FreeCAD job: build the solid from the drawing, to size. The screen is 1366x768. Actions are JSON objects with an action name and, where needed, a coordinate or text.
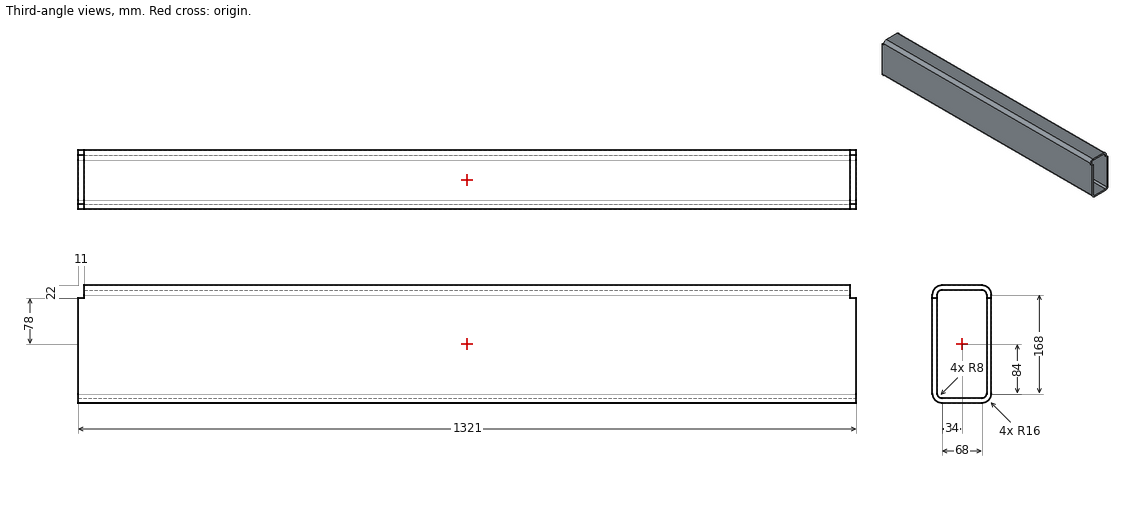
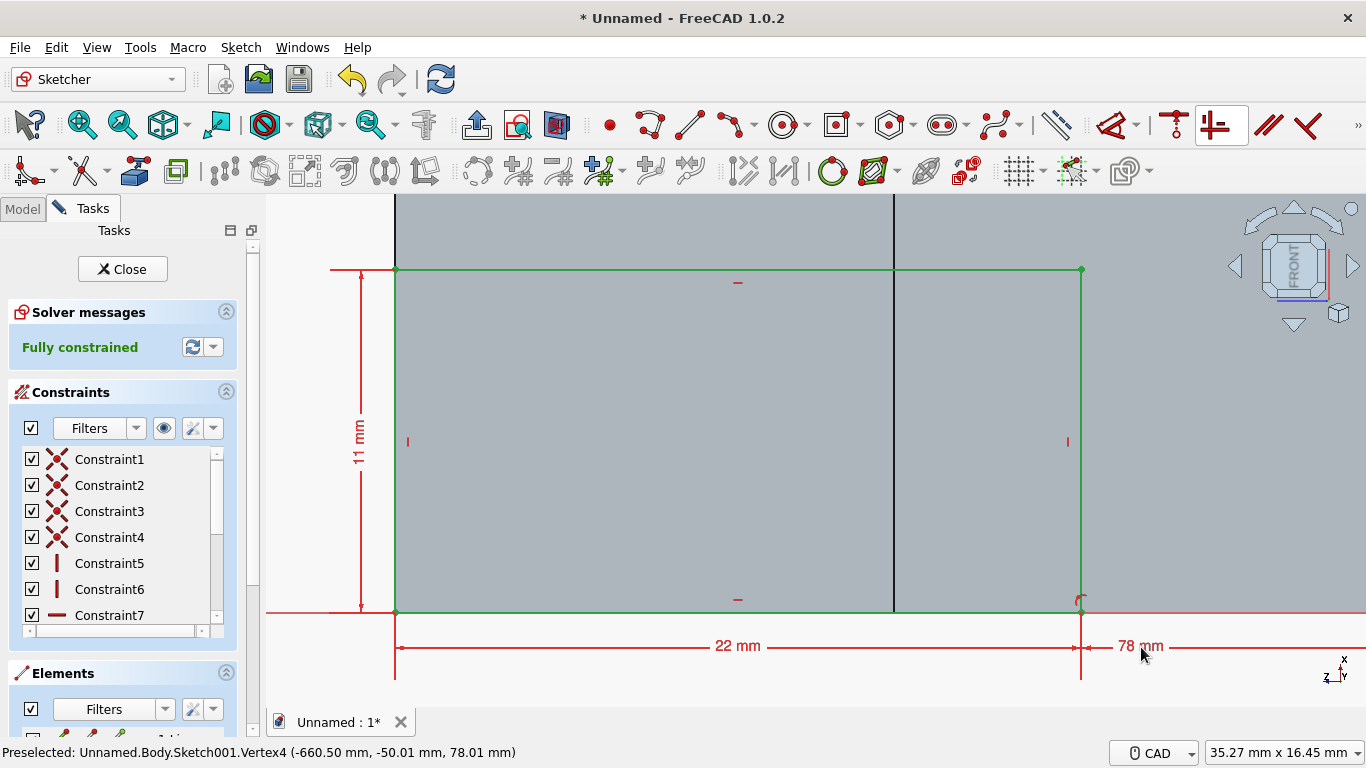
{"action": "left_click", "coordinate": [123, 269]}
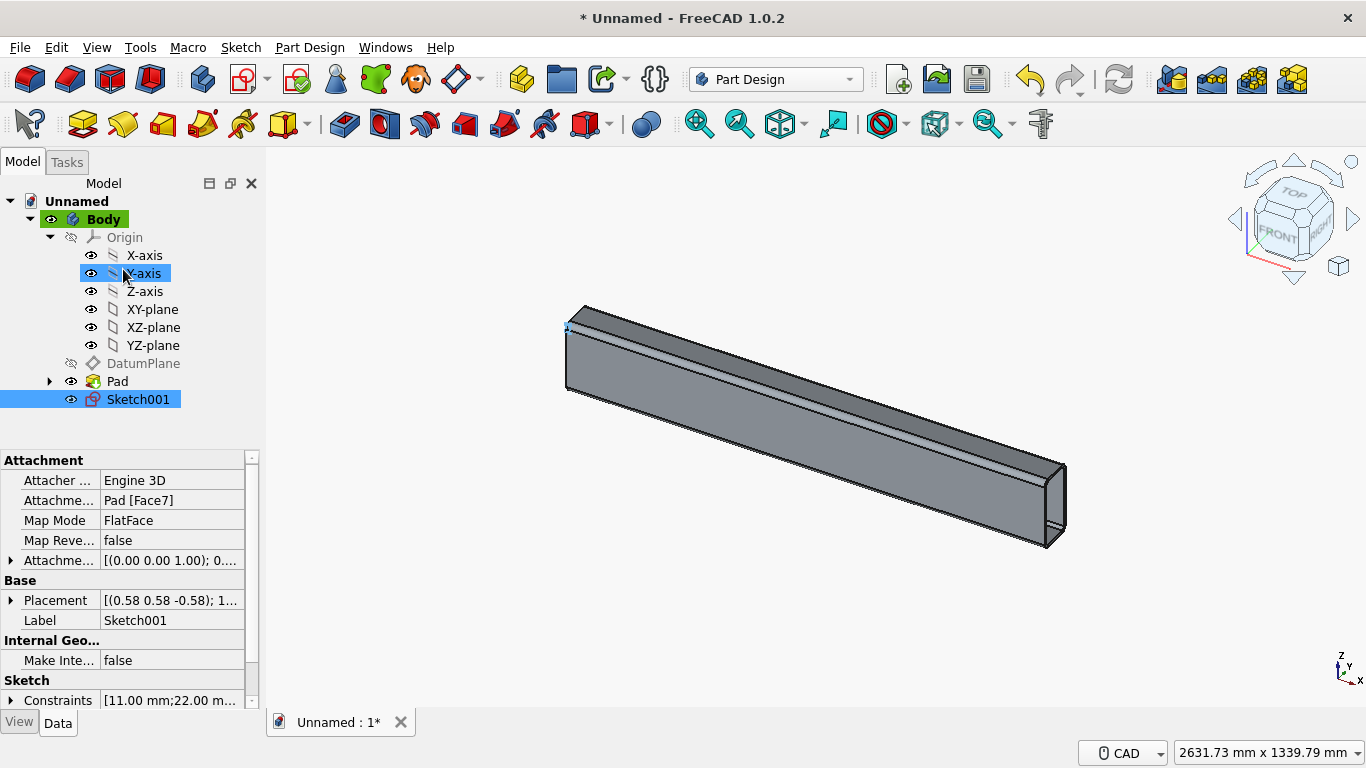
{"action": "left_click", "coordinate": [346, 124]}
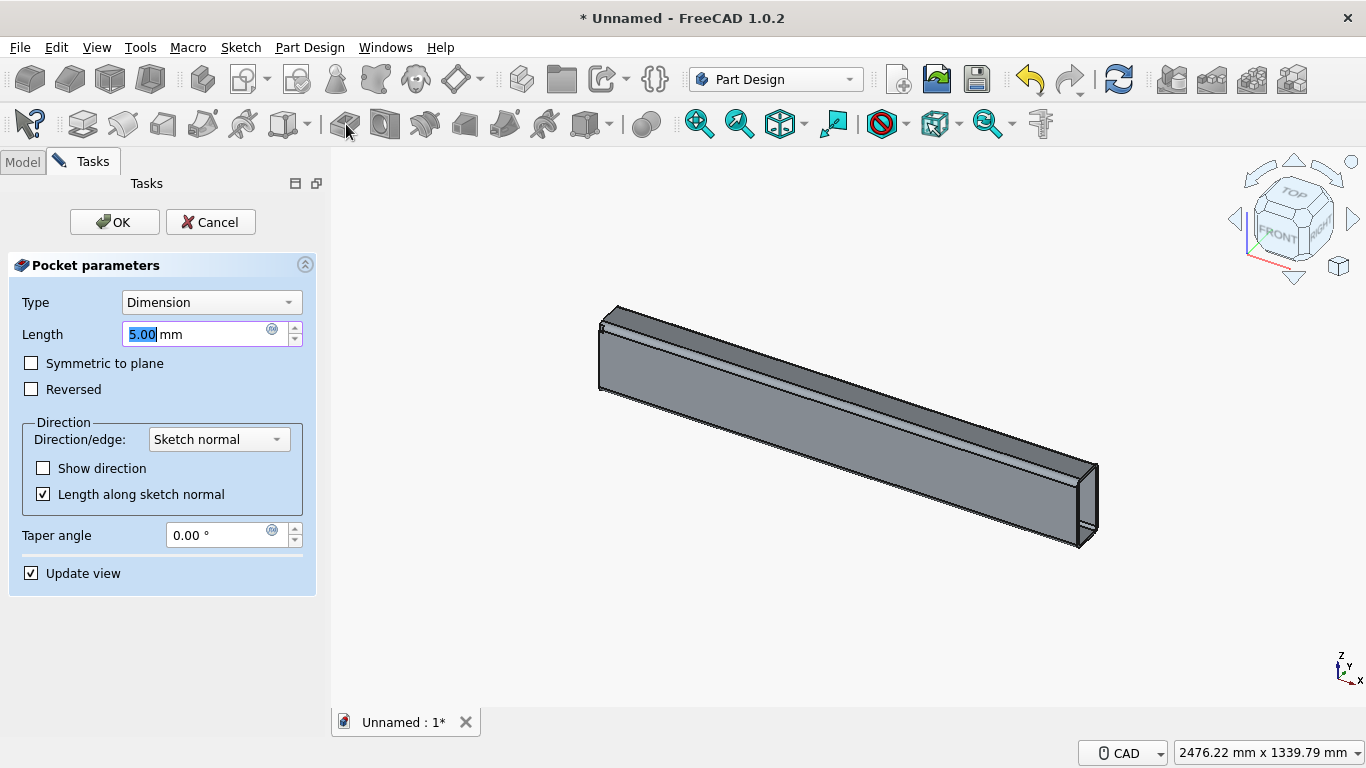
{"action": "left_click", "coordinate": [212, 302]}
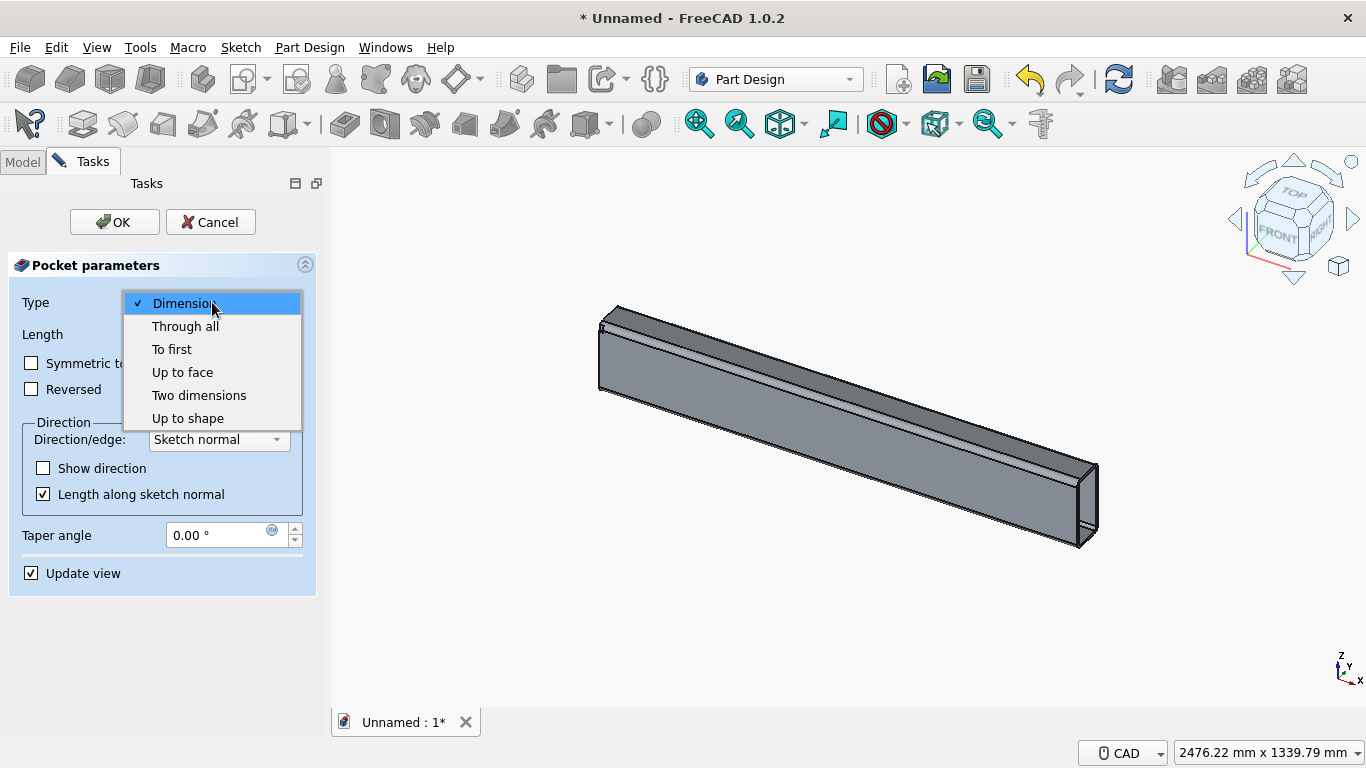
{"action": "left_click", "coordinate": [212, 326]}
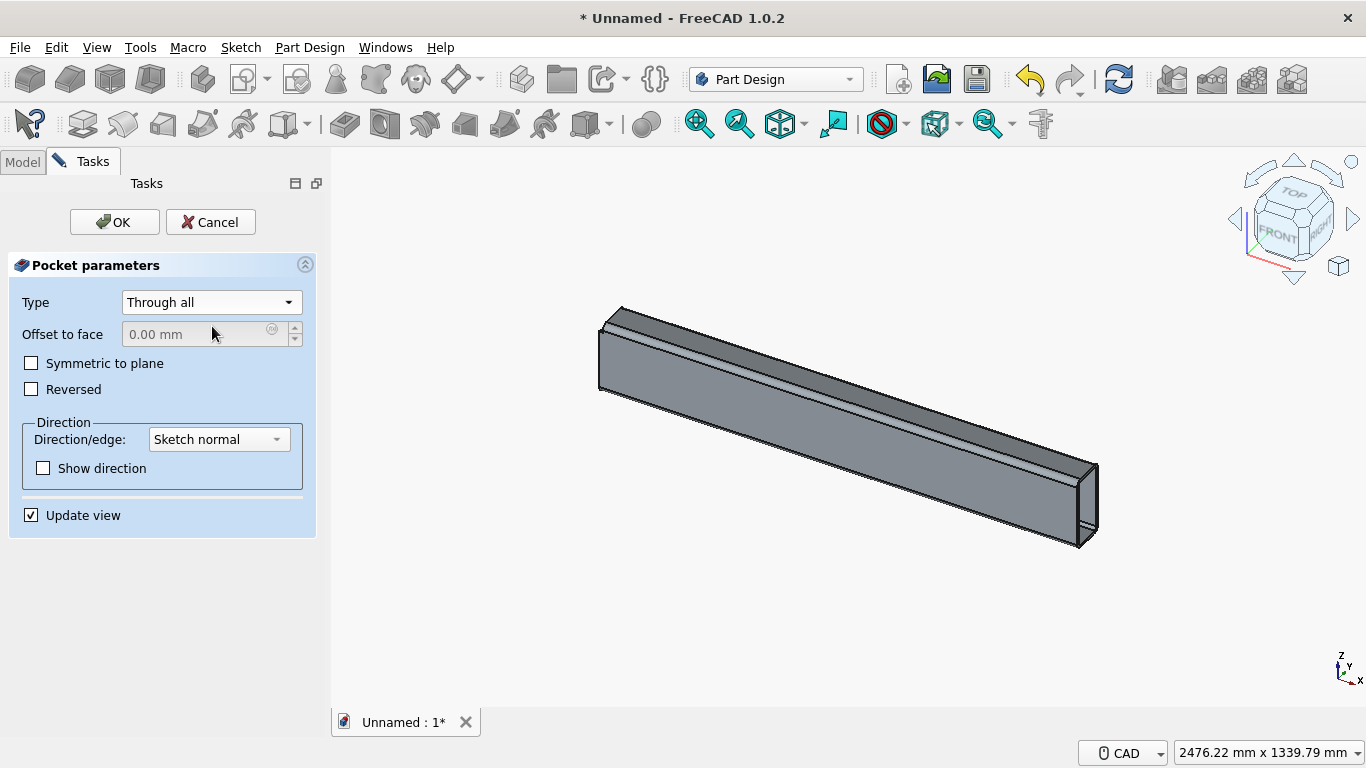
{"action": "left_click", "coordinate": [115, 222]}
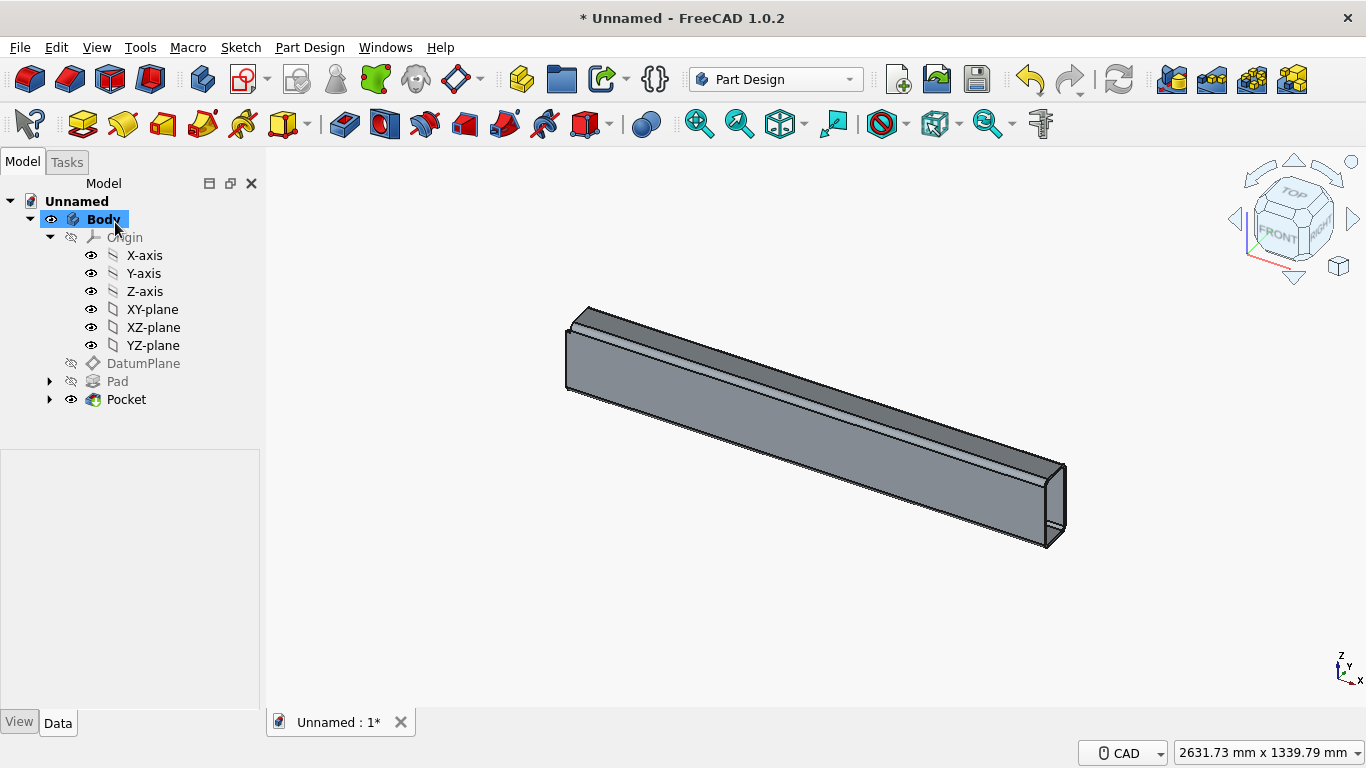
{"action": "left_click", "coordinate": [116, 399]}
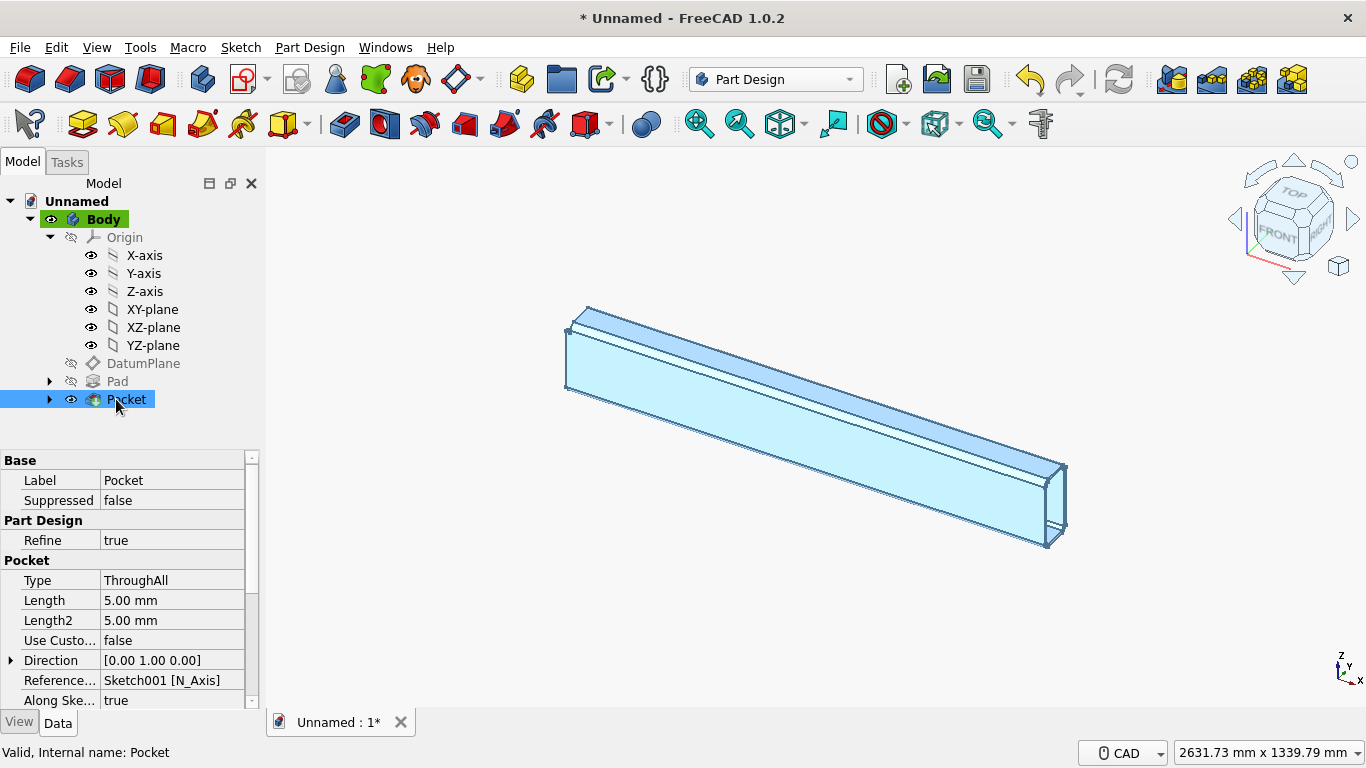
{"action": "left_click", "coordinate": [1172, 80]}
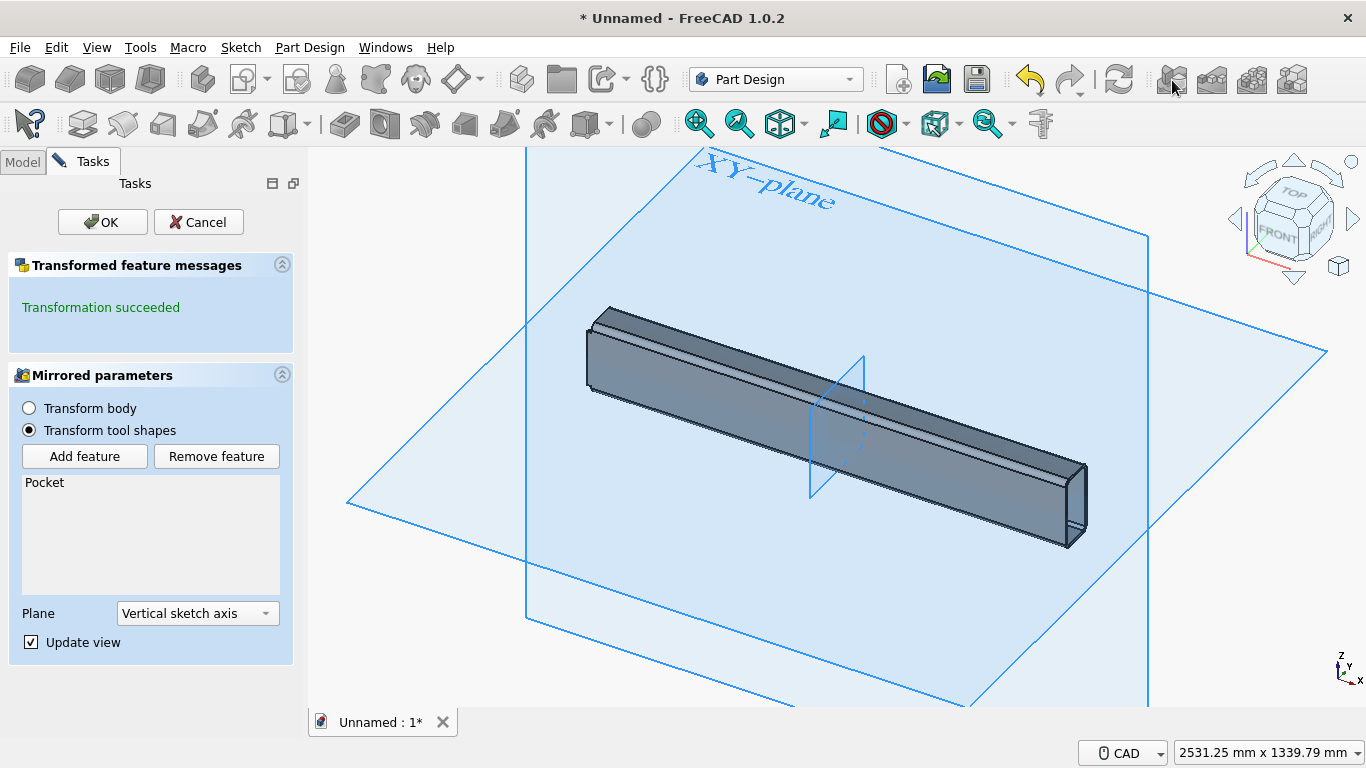
{"action": "left_click", "coordinate": [198, 614]}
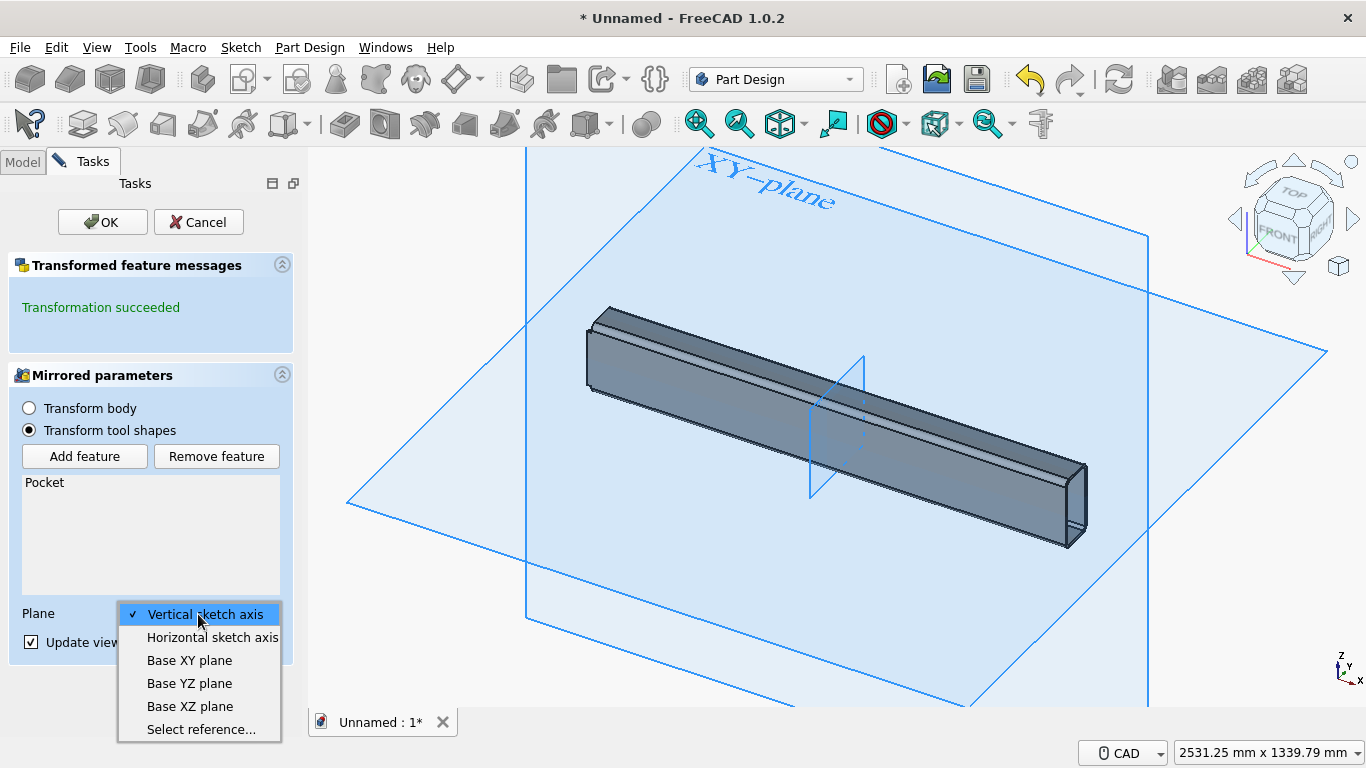
{"action": "left_click", "coordinate": [198, 684]}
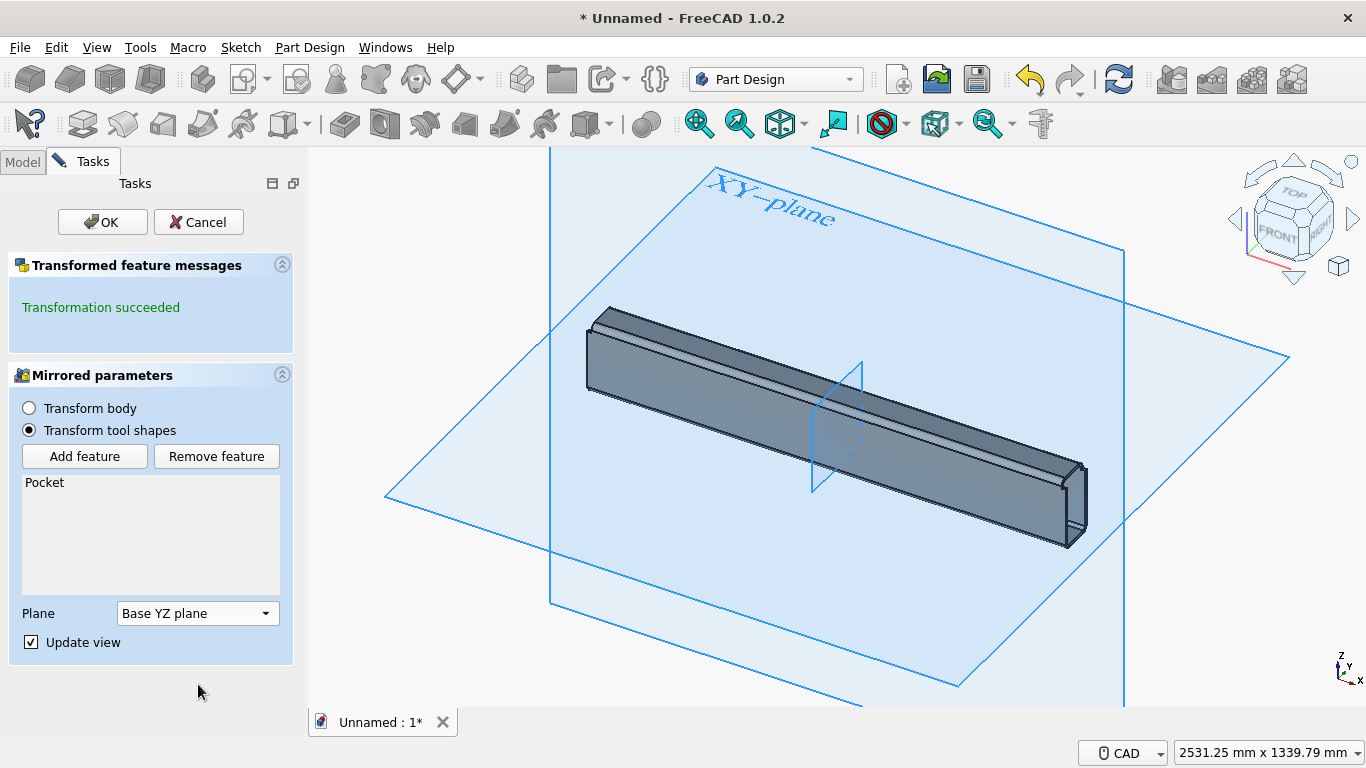
{"action": "left_click", "coordinate": [103, 222]}